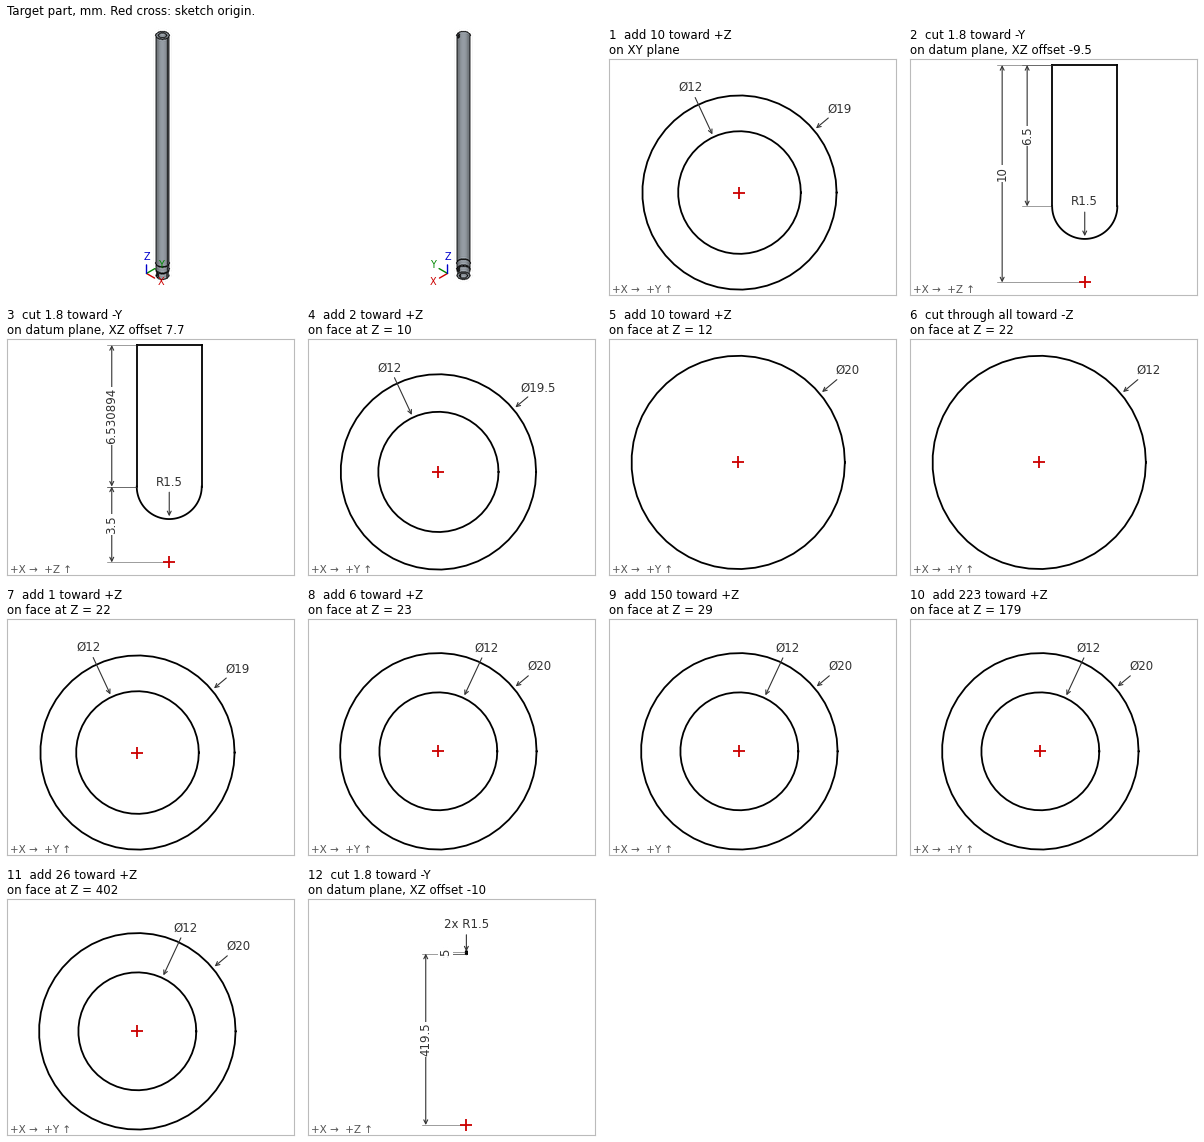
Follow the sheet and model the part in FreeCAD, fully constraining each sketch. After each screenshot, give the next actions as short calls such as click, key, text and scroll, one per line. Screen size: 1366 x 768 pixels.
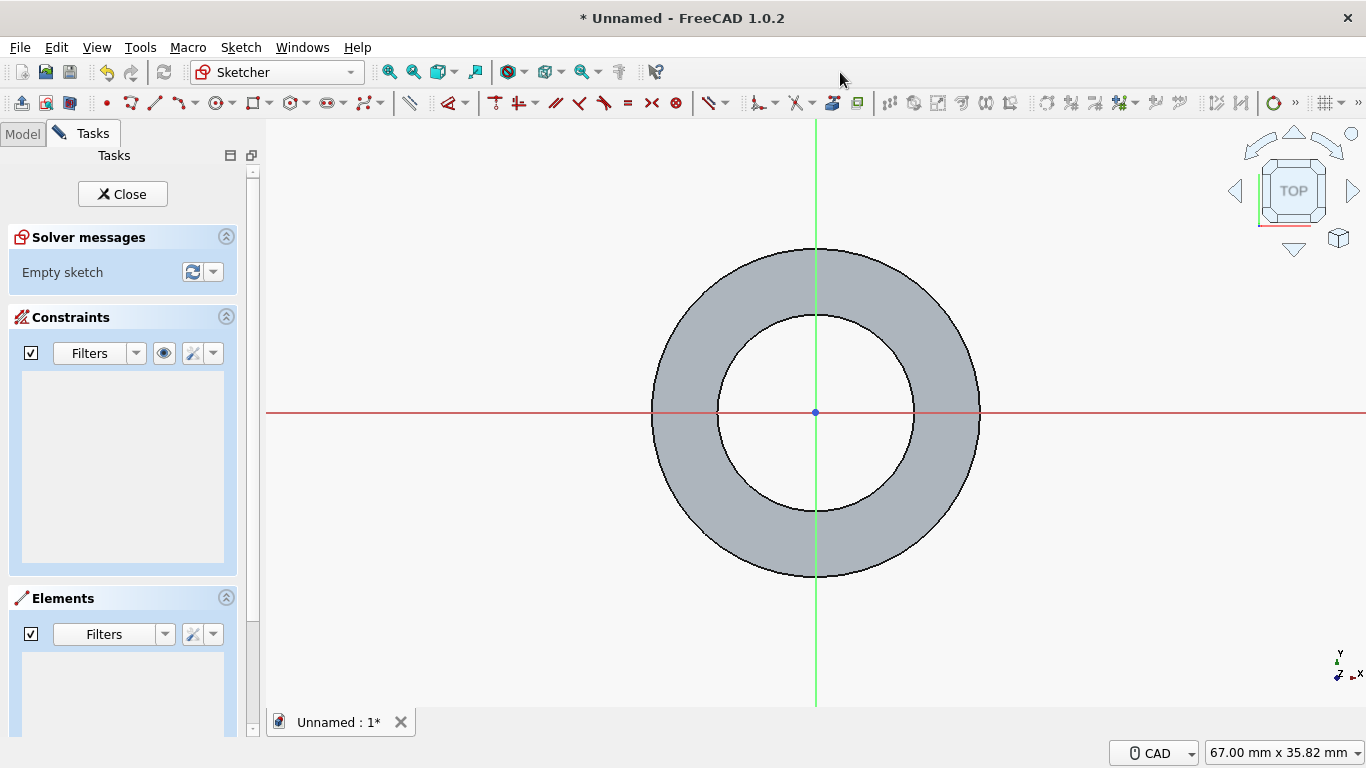
click(216, 104)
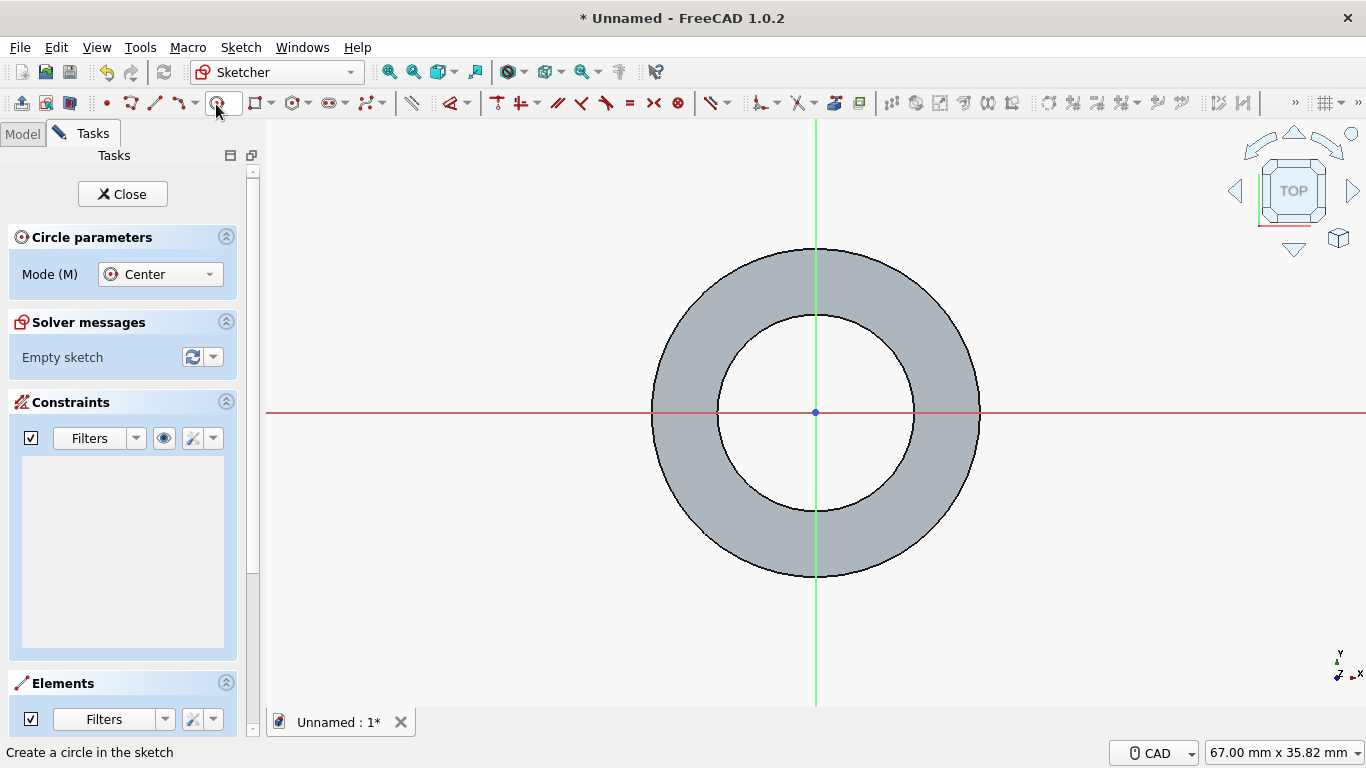
click(816, 413)
click(926, 303)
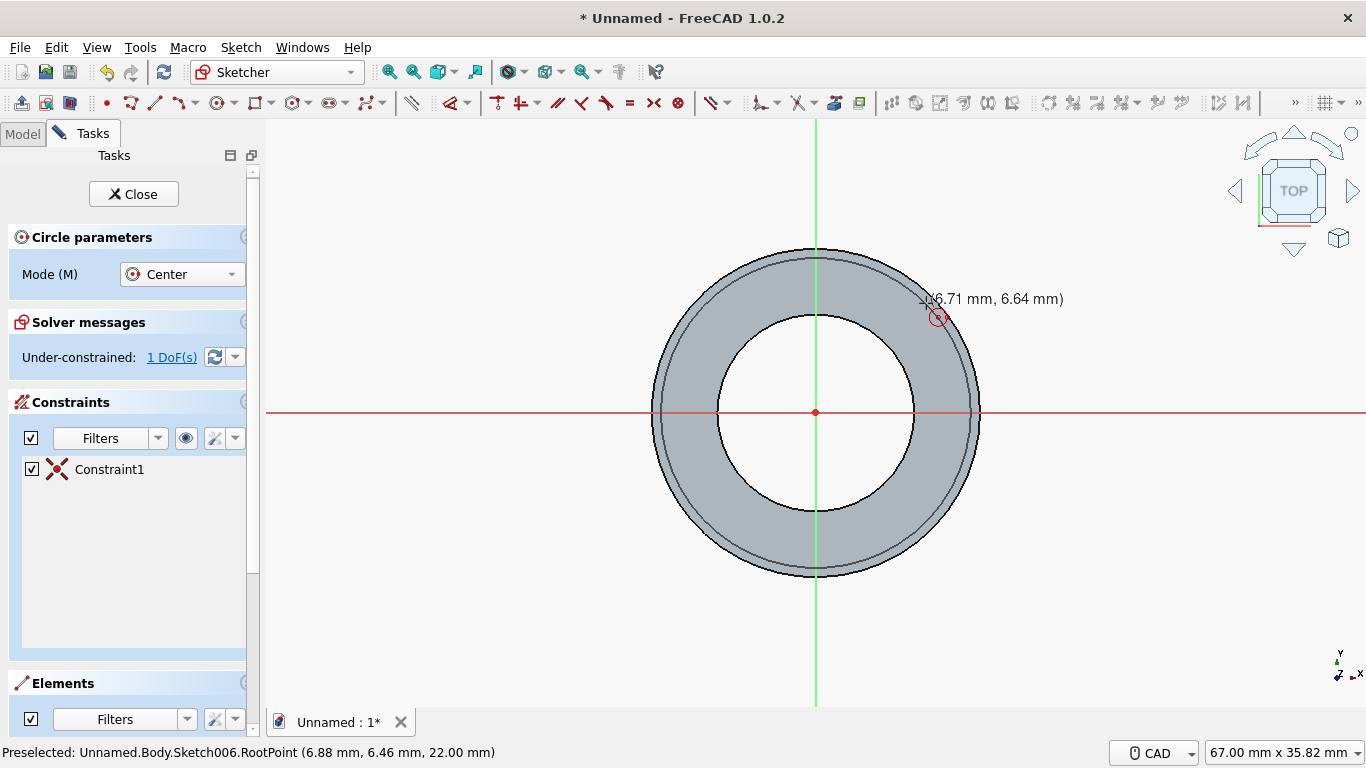
click(816, 413)
click(885, 343)
key(Escape)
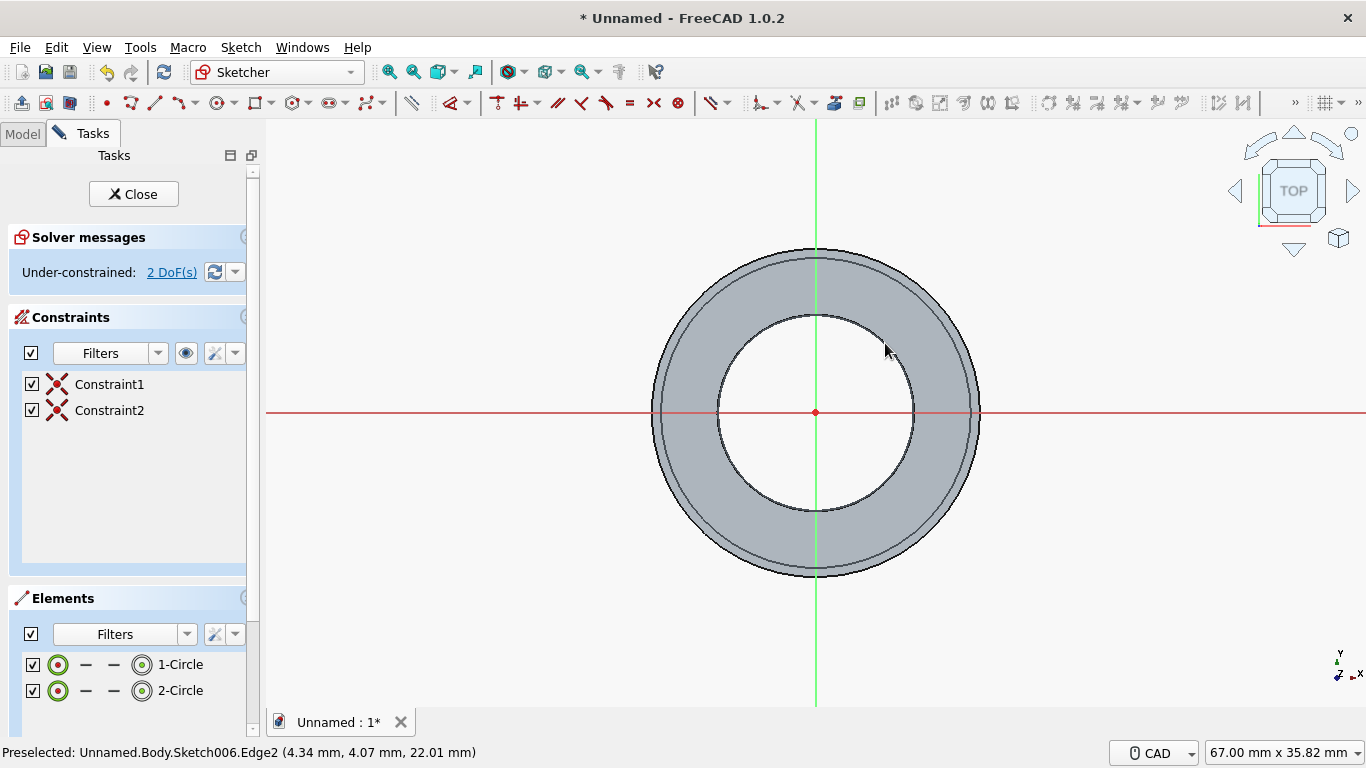
click(450, 104)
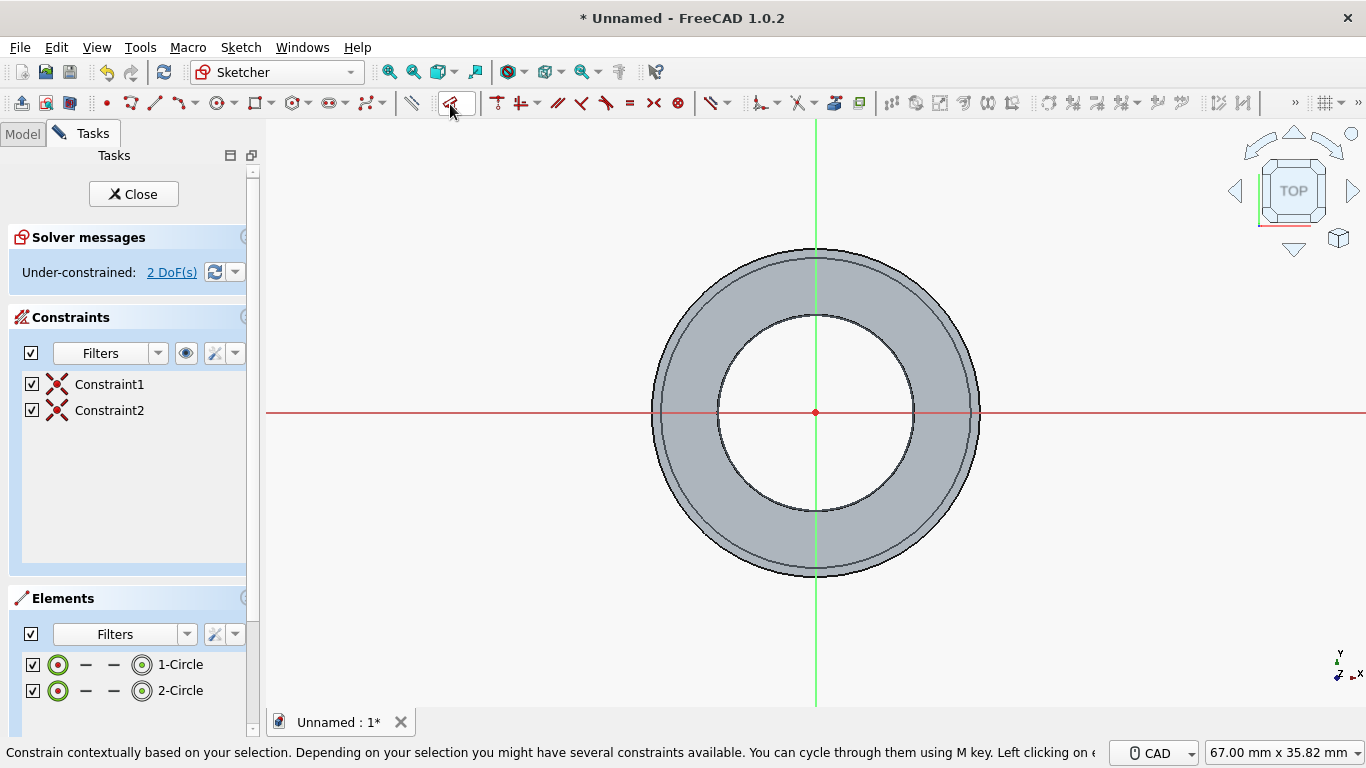
click(925, 303)
click(948, 280)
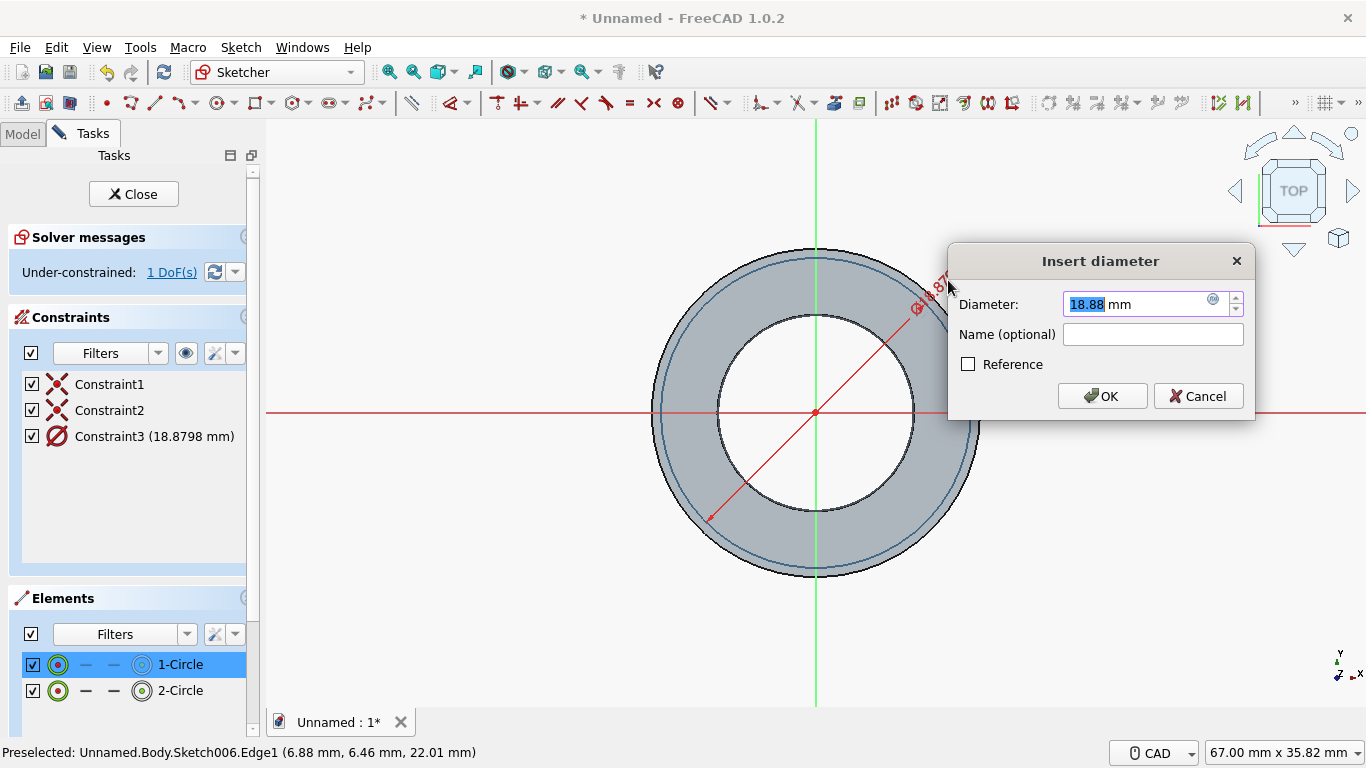
text(19)
key(Return)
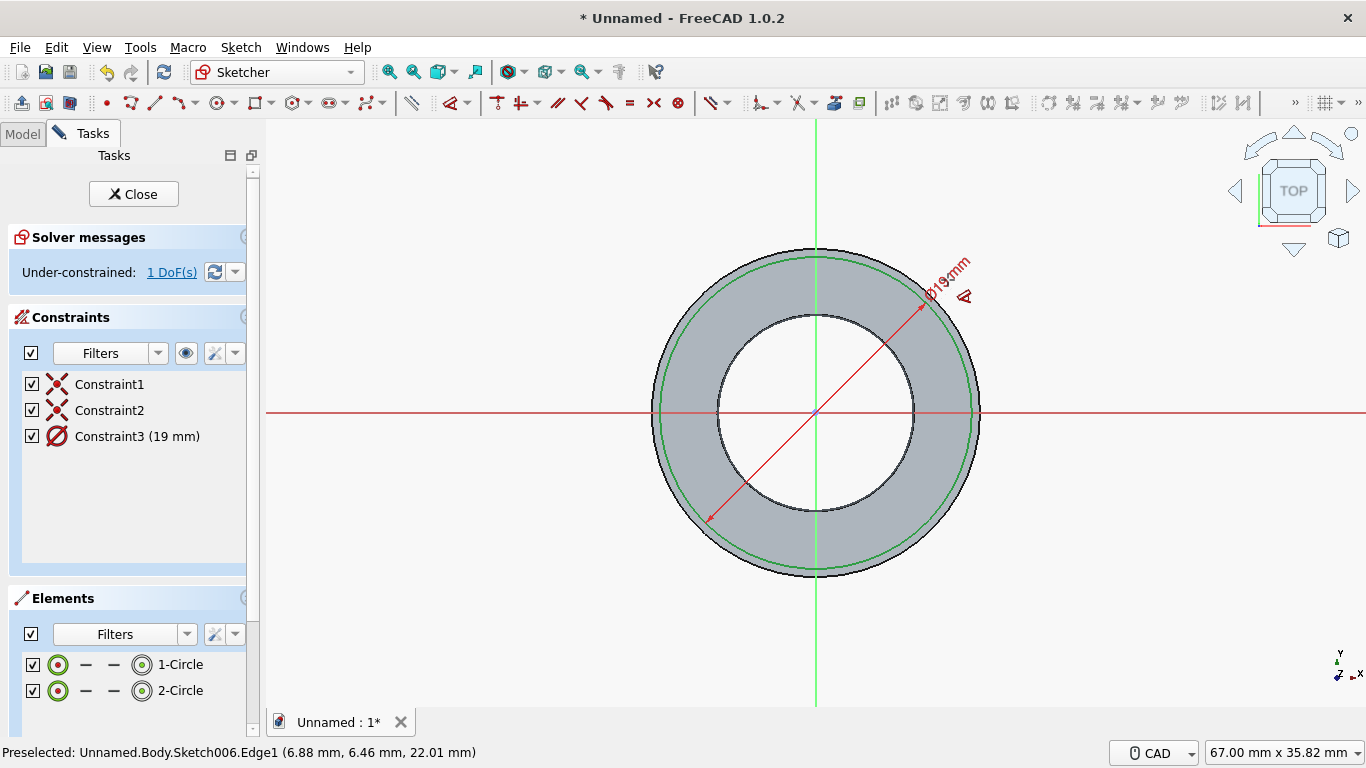
click(885, 344)
click(908, 321)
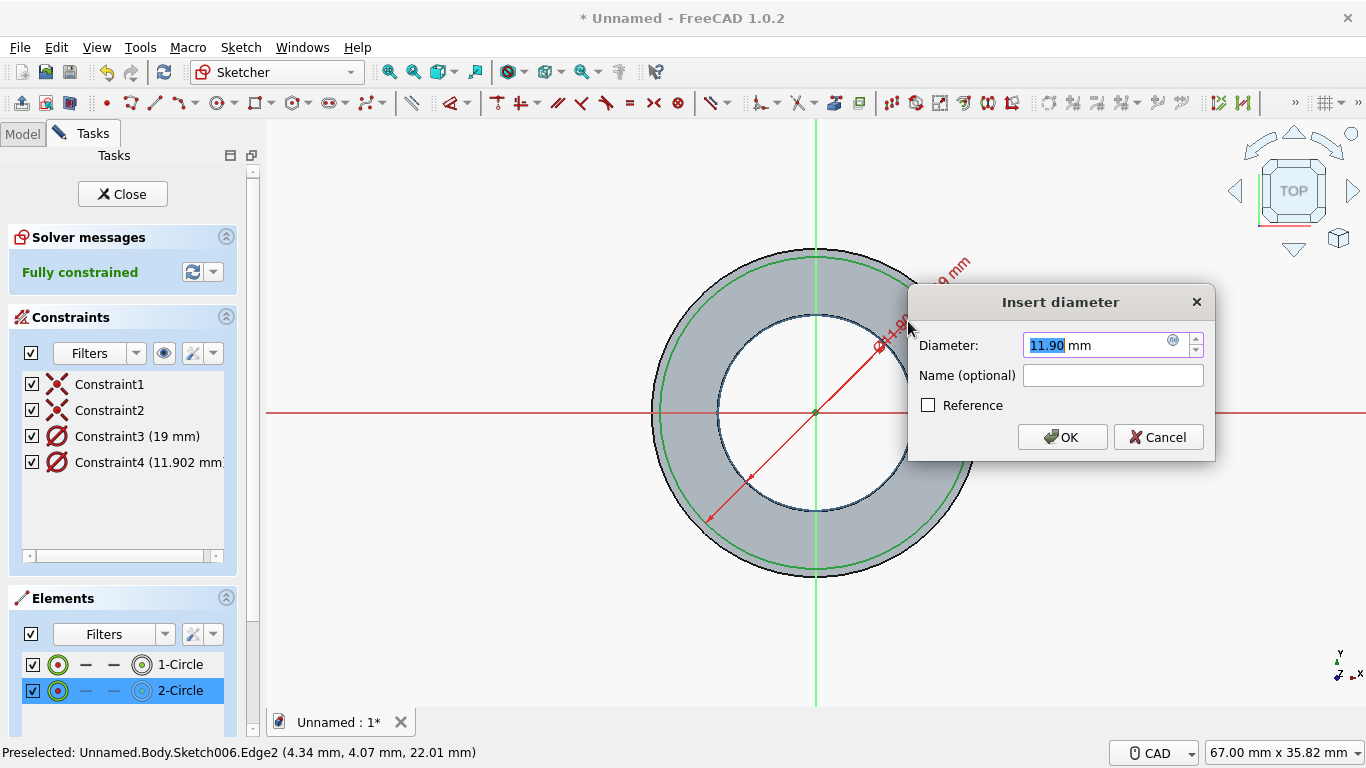
text(12)
key(Return)
key(Escape)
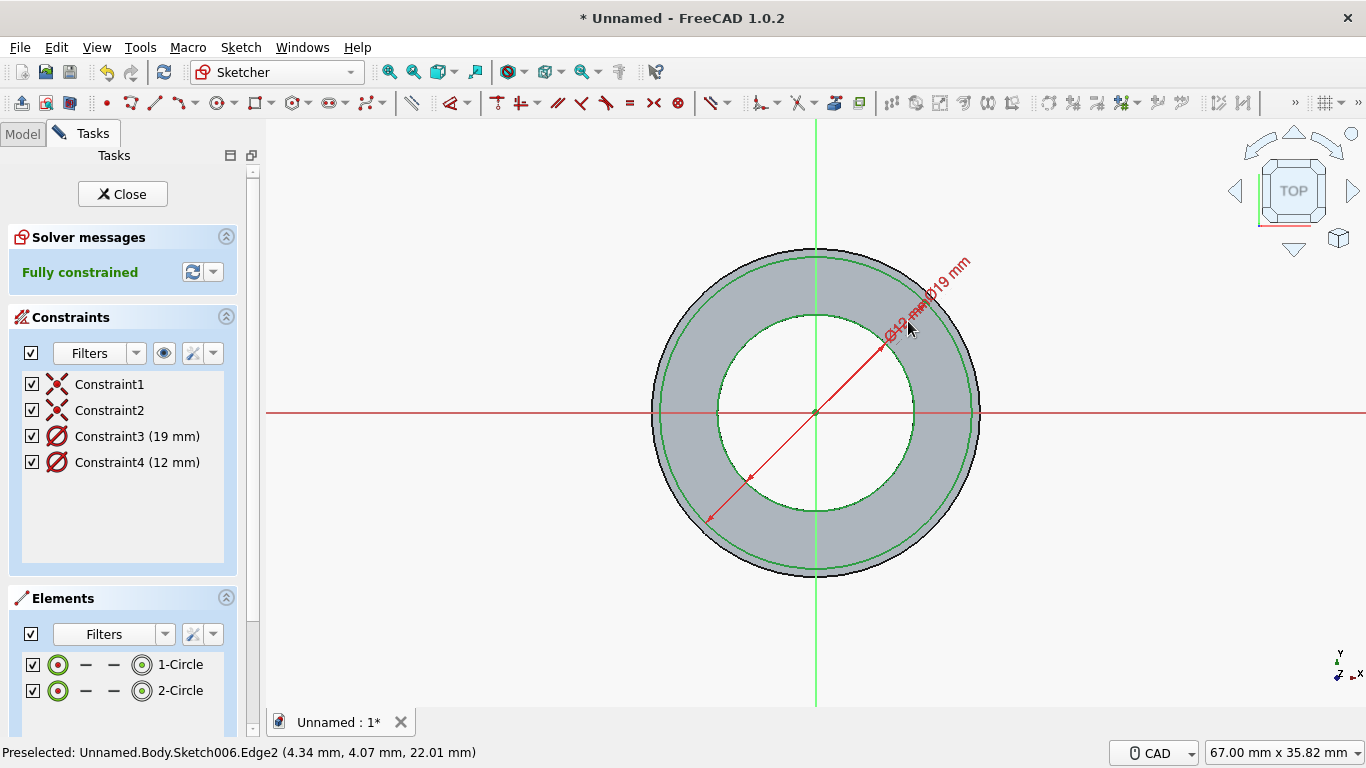
click(123, 194)